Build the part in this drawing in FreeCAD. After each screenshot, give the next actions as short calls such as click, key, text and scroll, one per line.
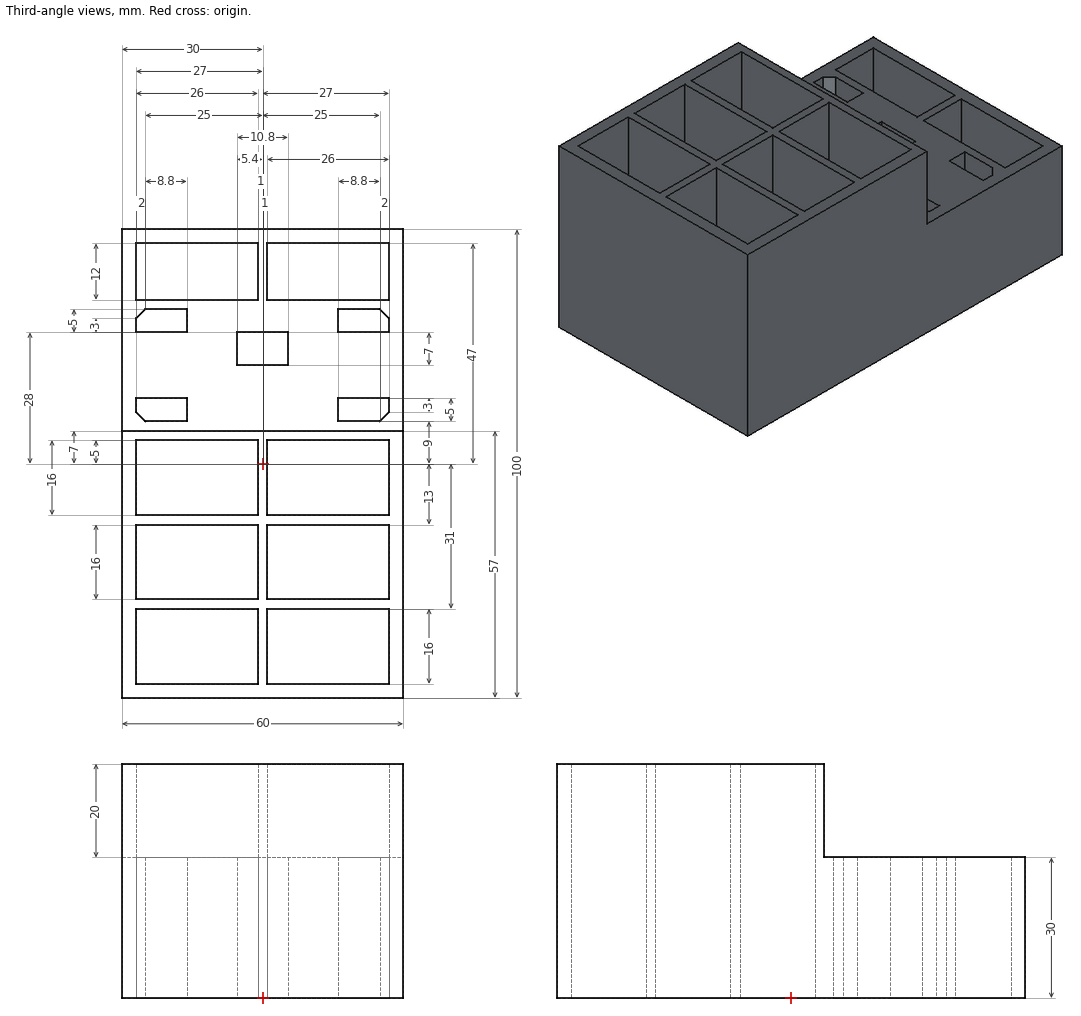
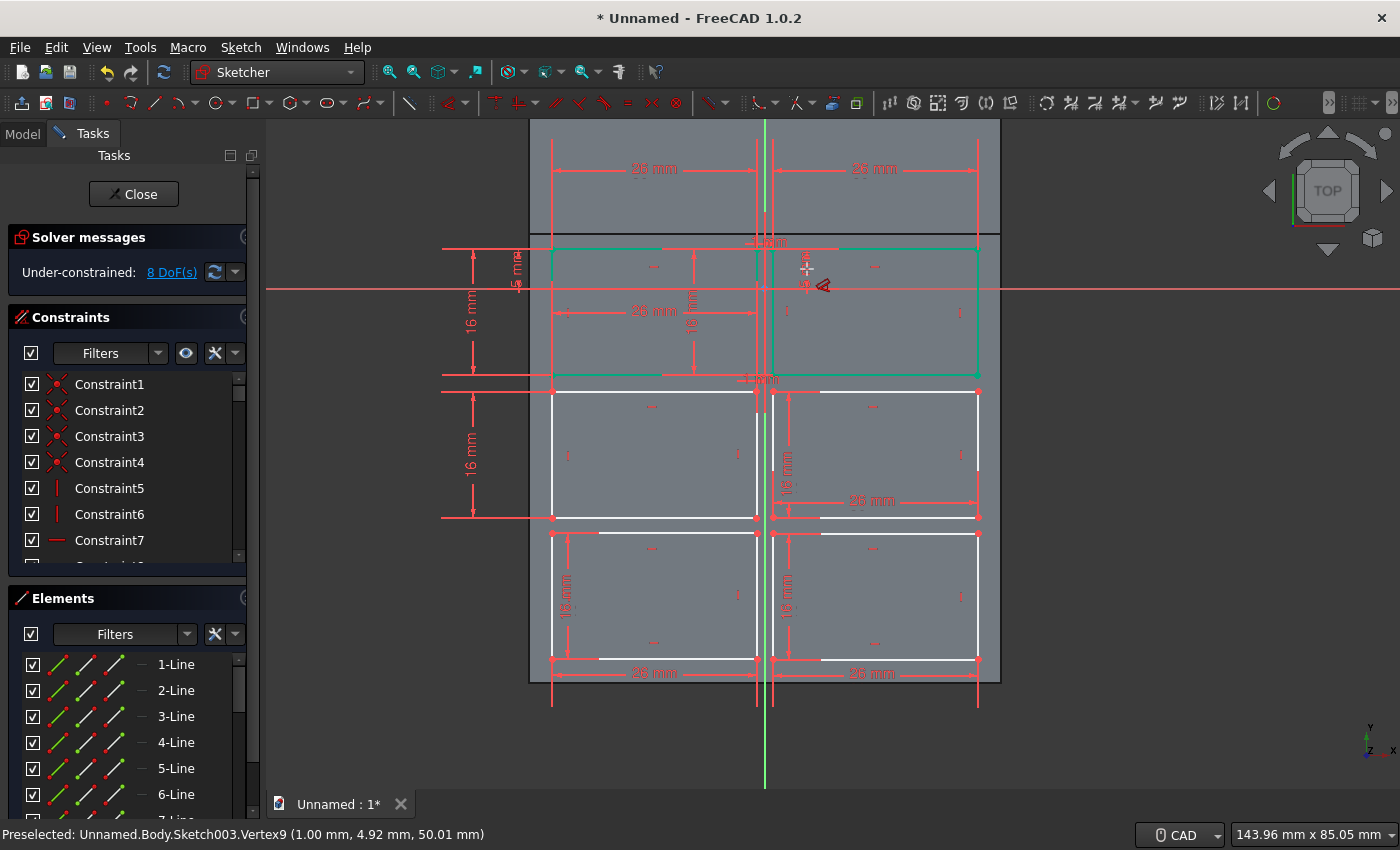
scroll(773, 392, up, 9)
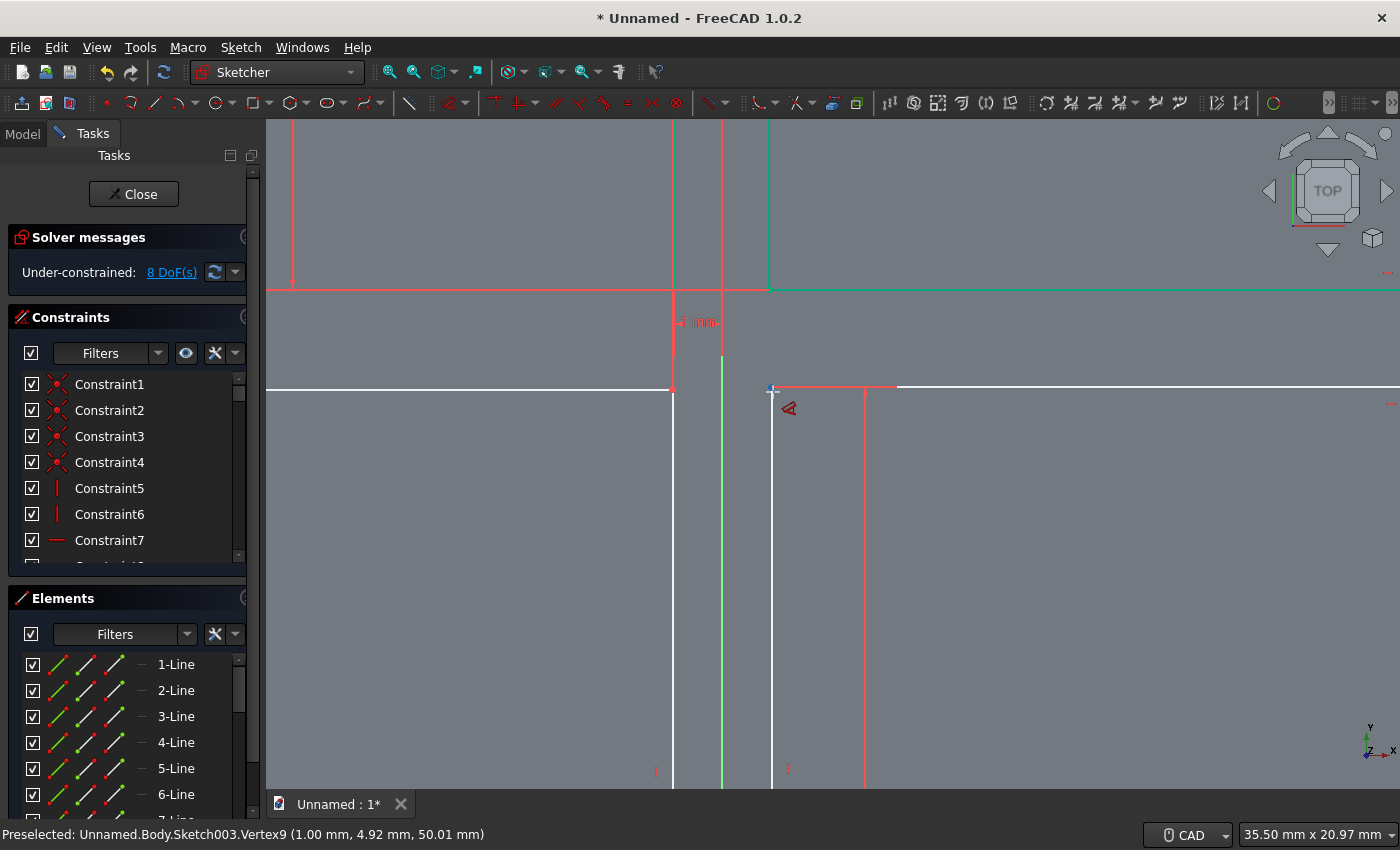
click(772, 387)
click(747, 421)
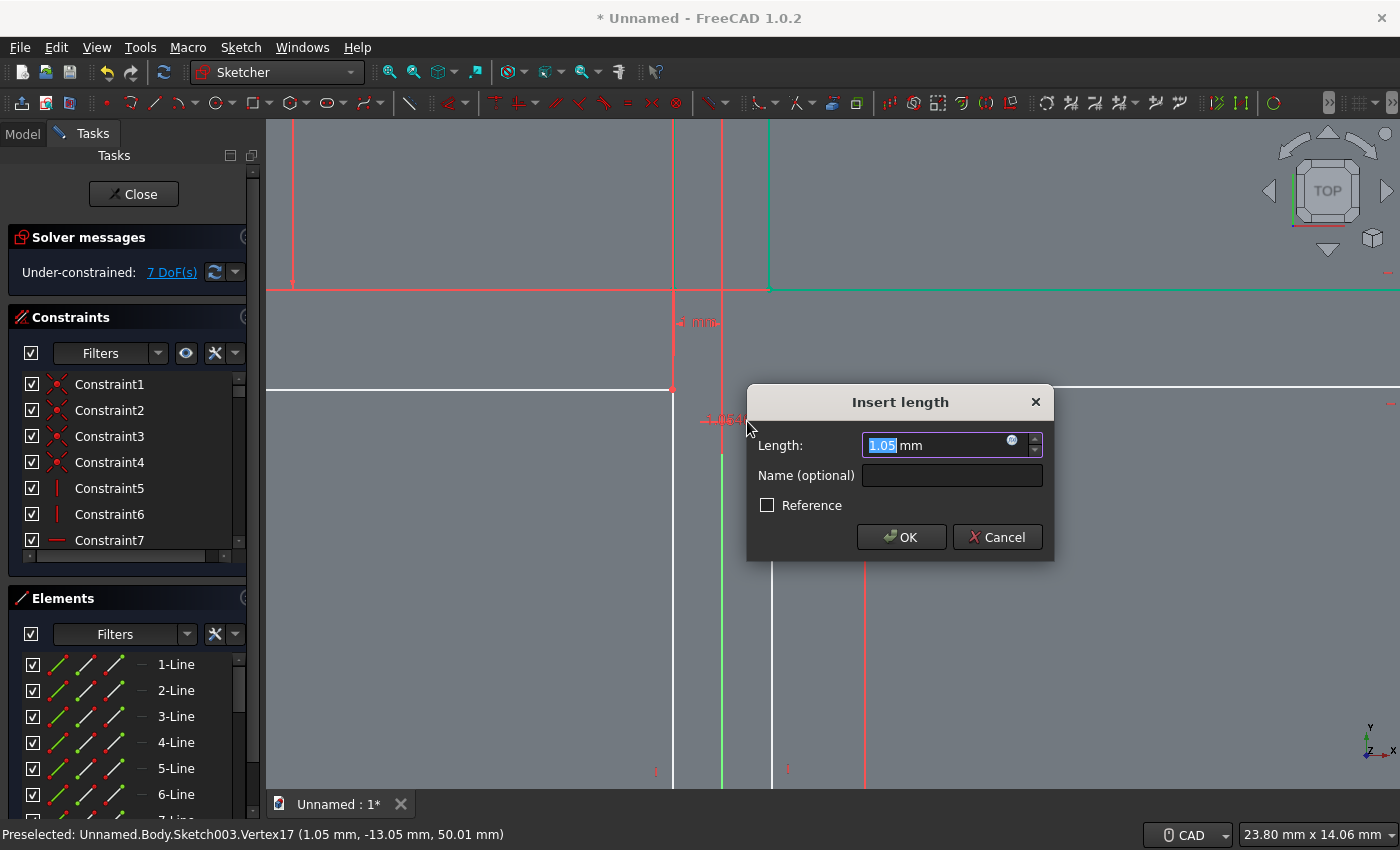
text(1)
key(Return)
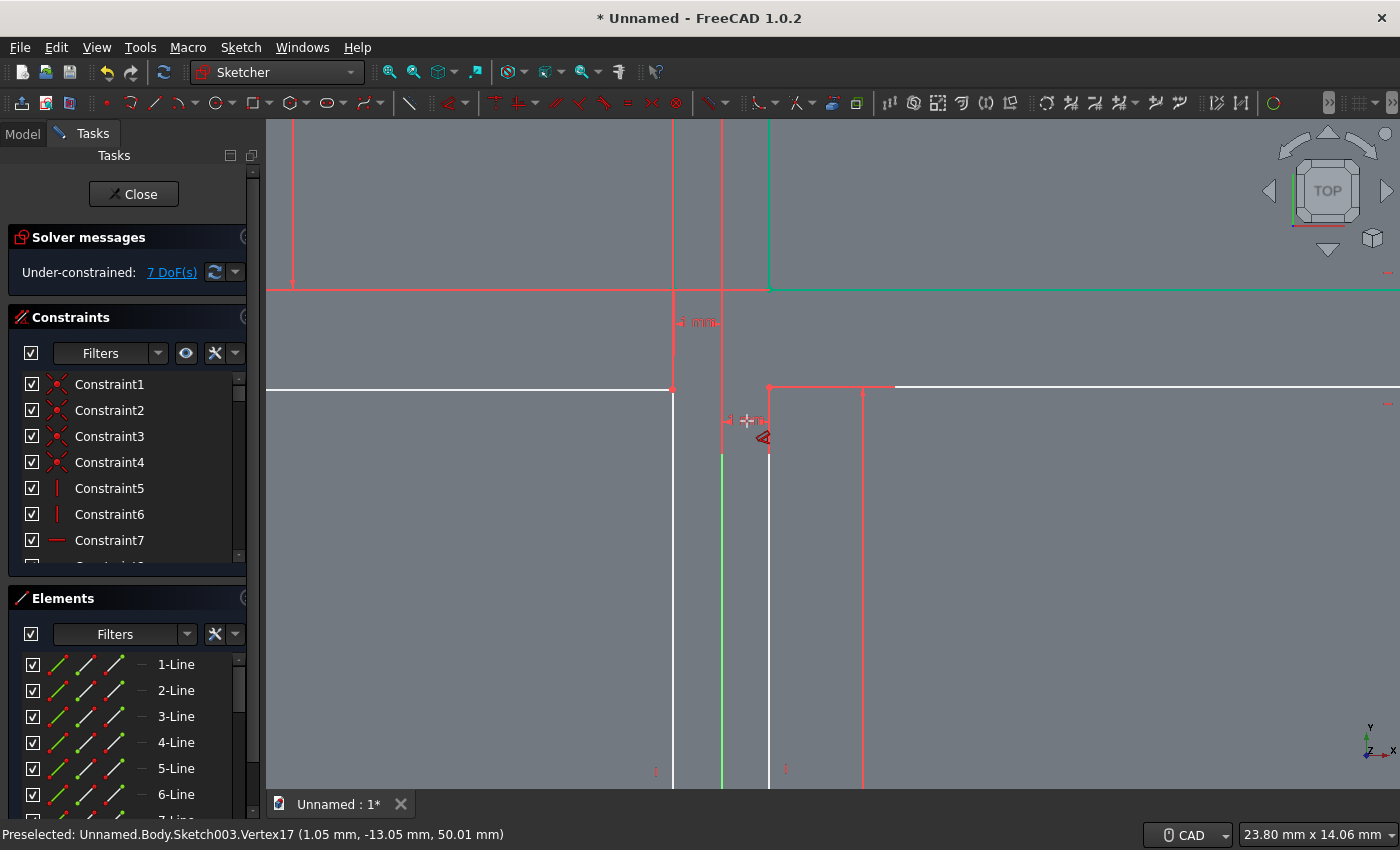
scroll(773, 392, down, 9)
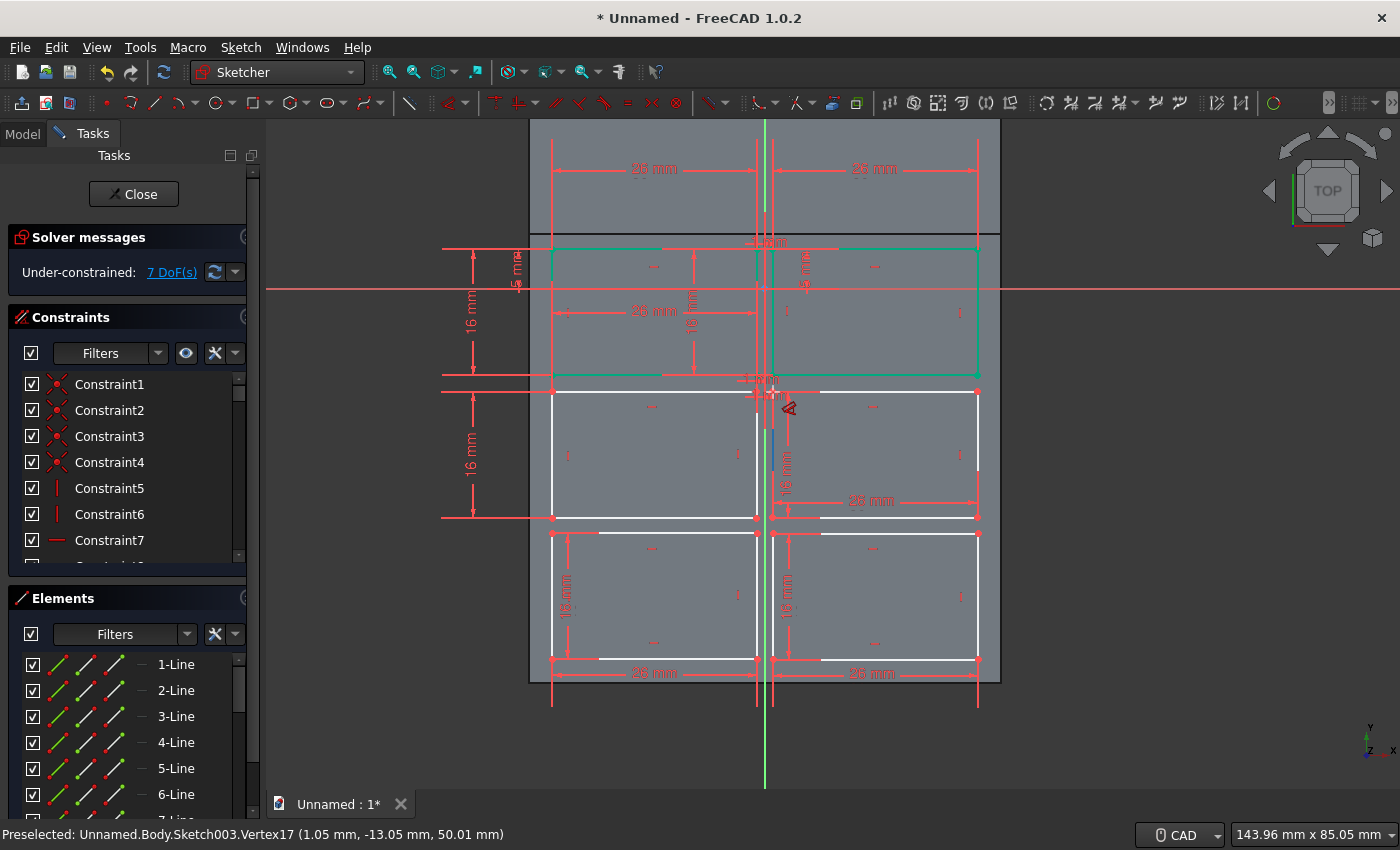
scroll(773, 534, up, 9)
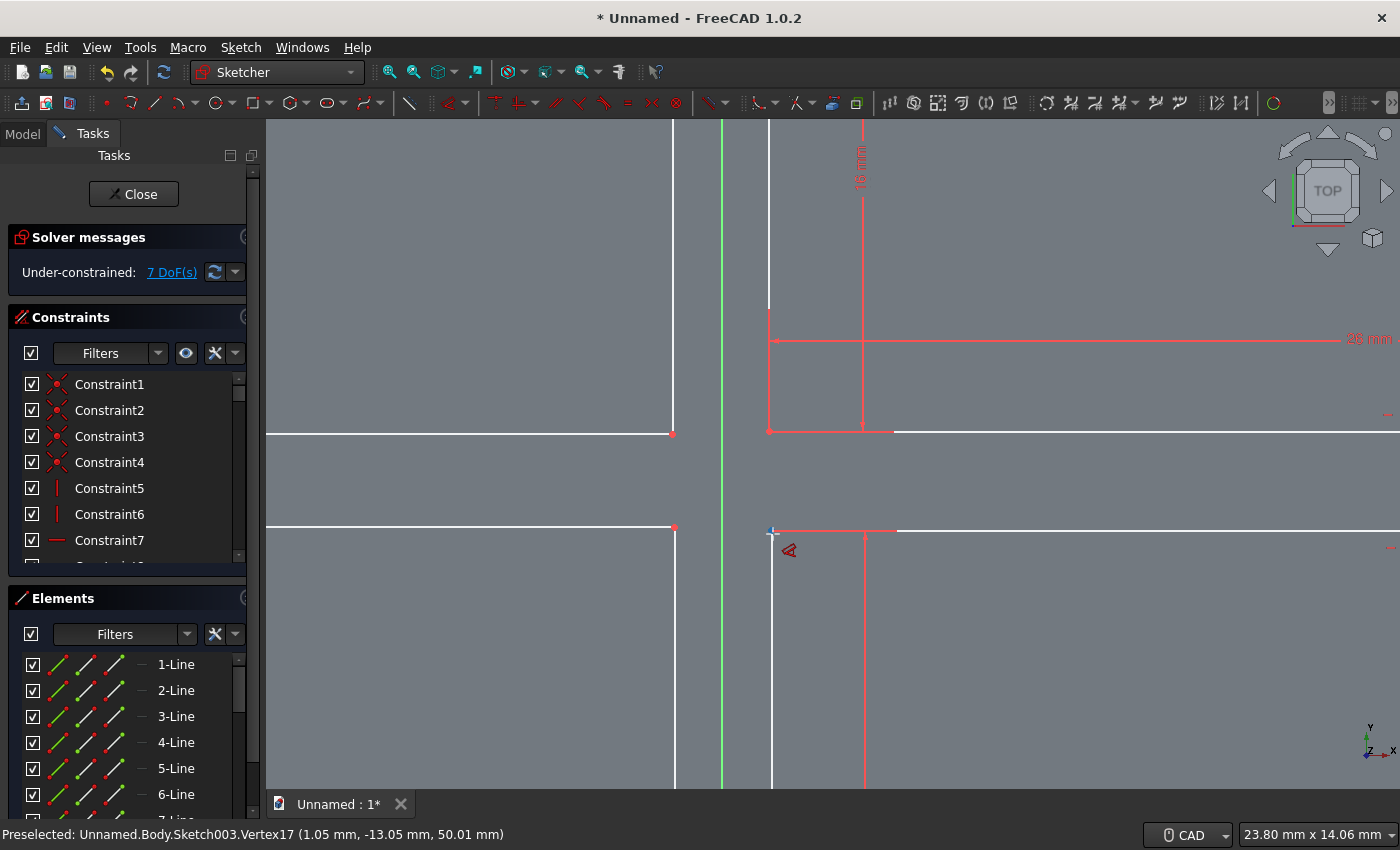
click(772, 531)
click(747, 565)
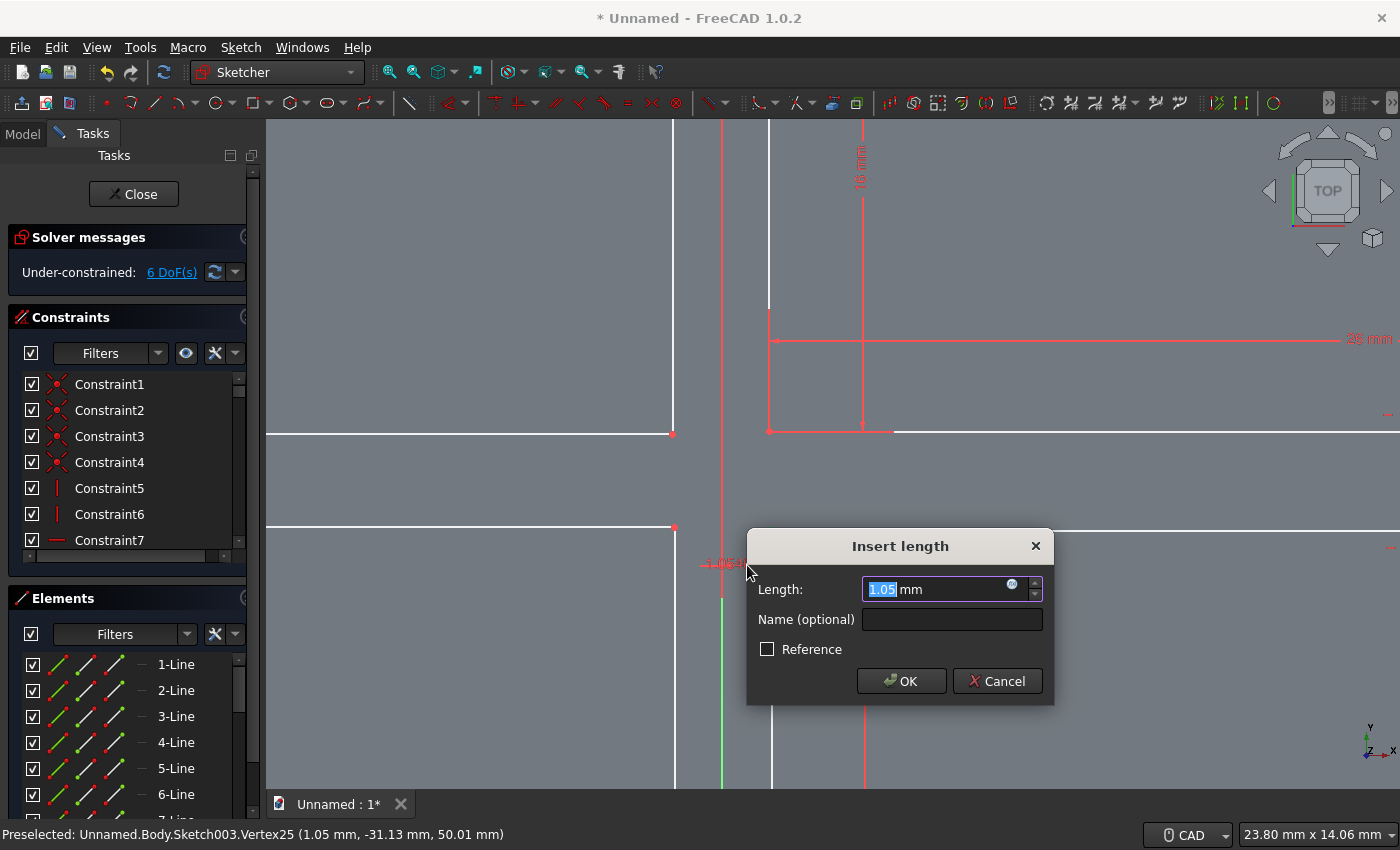
text(1)
key(Return)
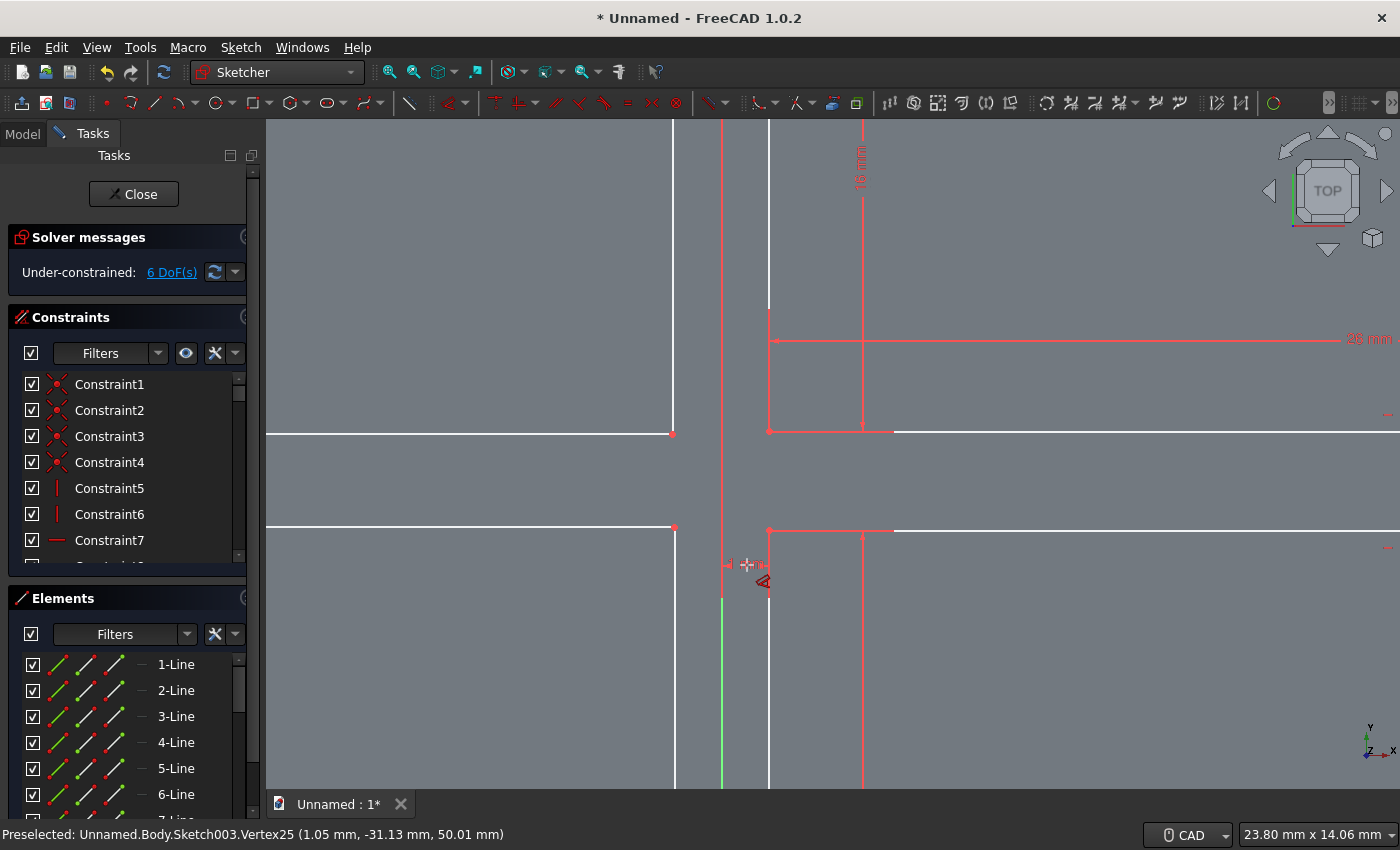
click(673, 434)
click(697, 468)